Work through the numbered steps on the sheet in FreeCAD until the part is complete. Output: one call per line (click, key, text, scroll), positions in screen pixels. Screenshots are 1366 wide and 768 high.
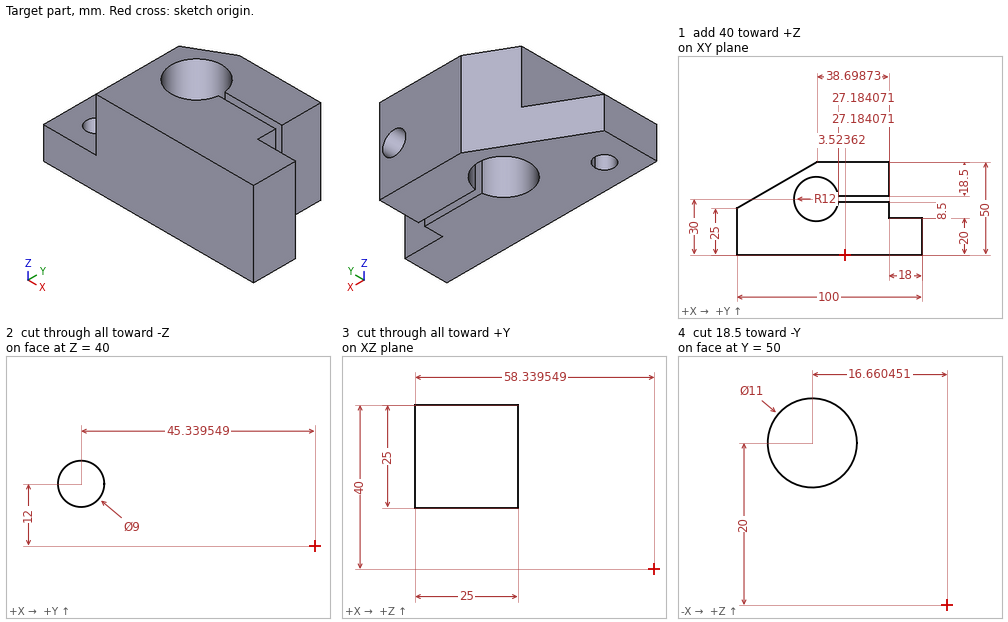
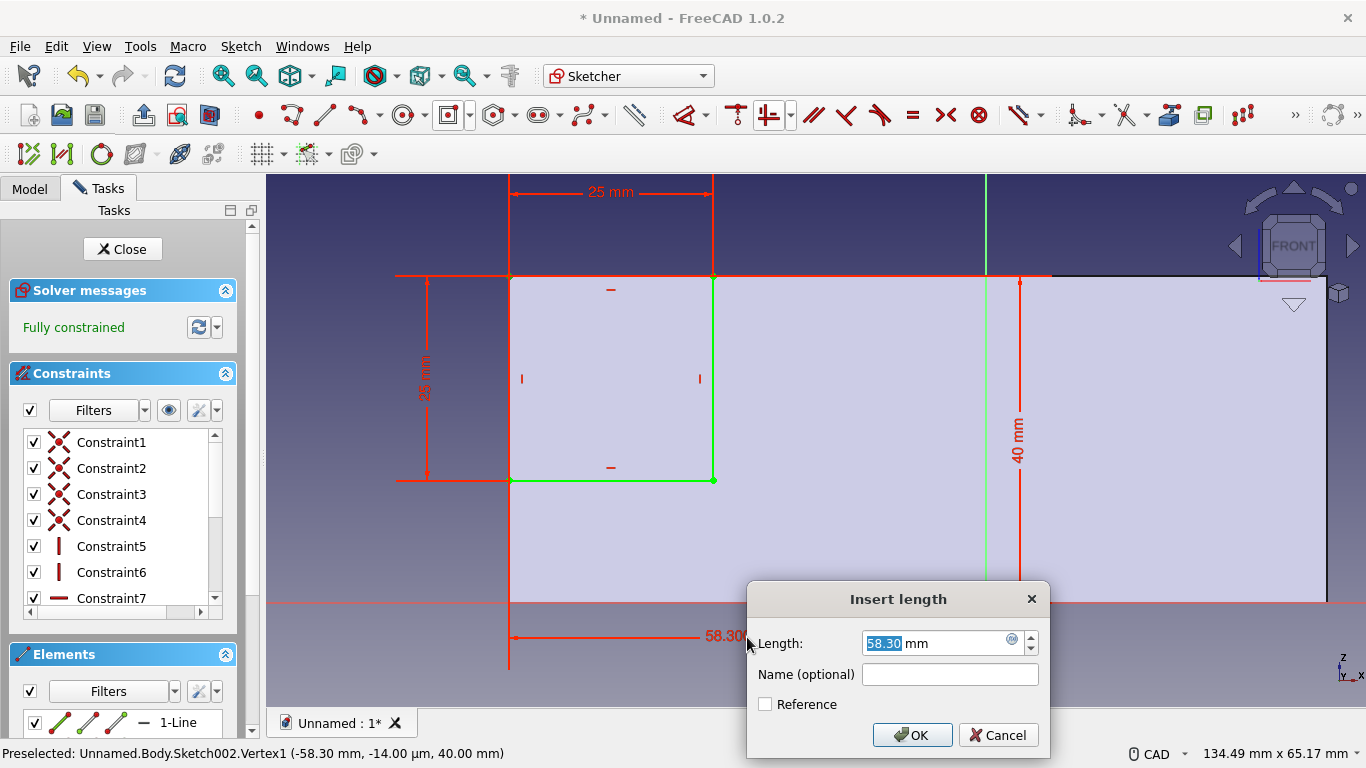
text(58.339549)
key(Return)
key(Escape)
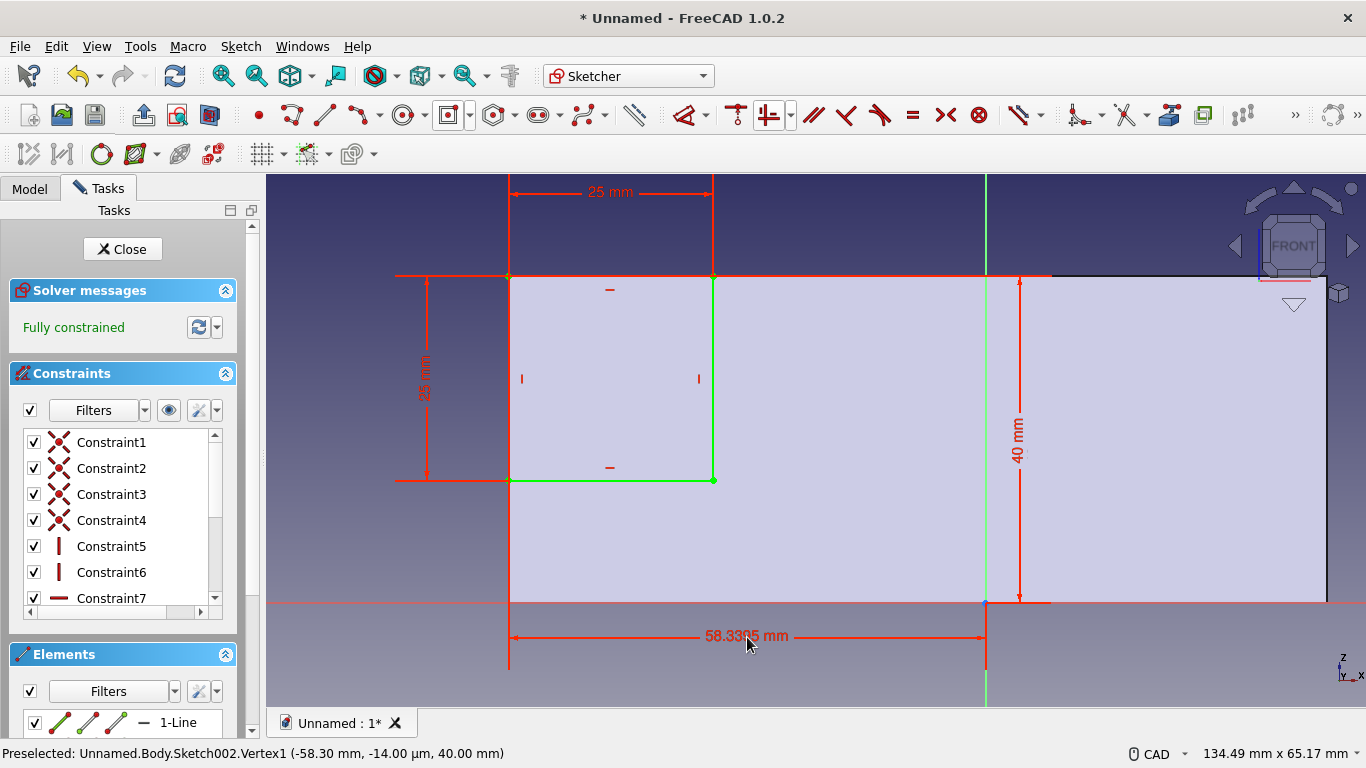
click(123, 249)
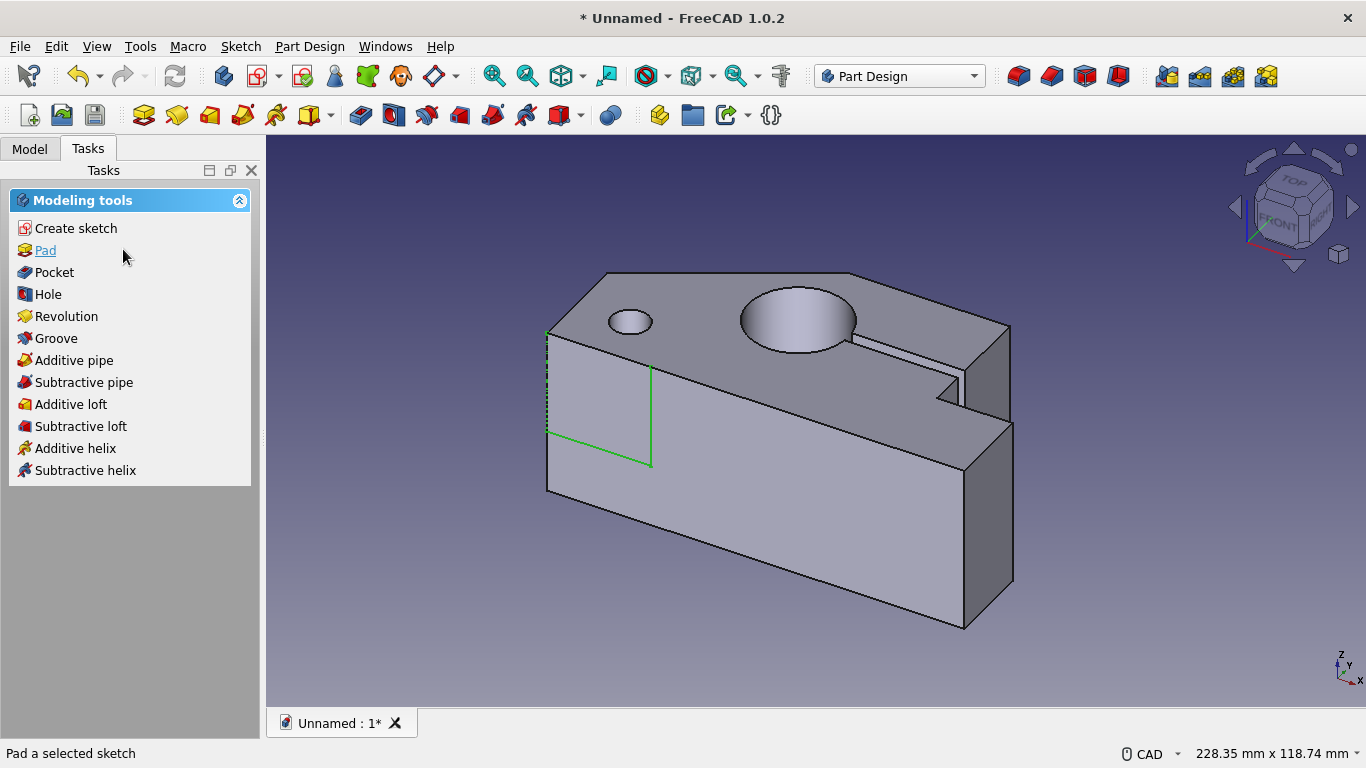
click(361, 116)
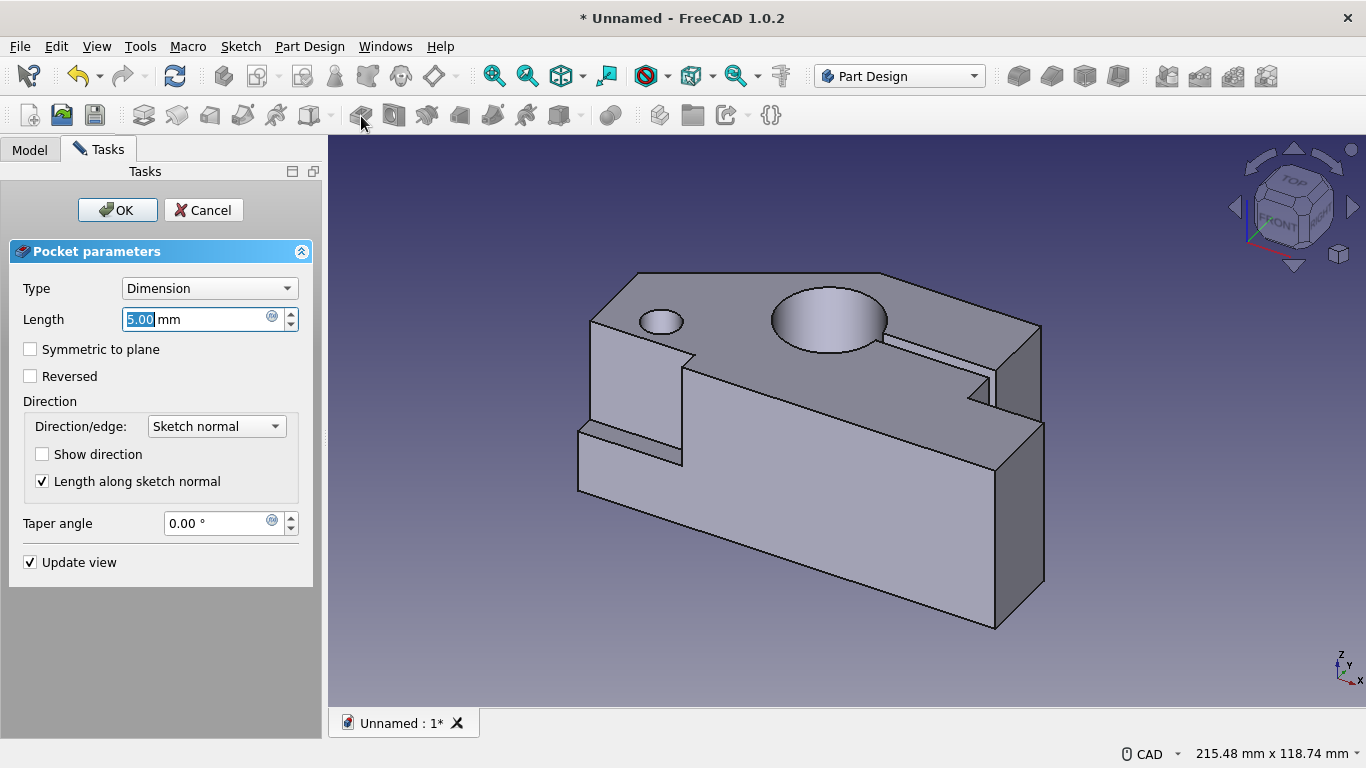
click(210, 288)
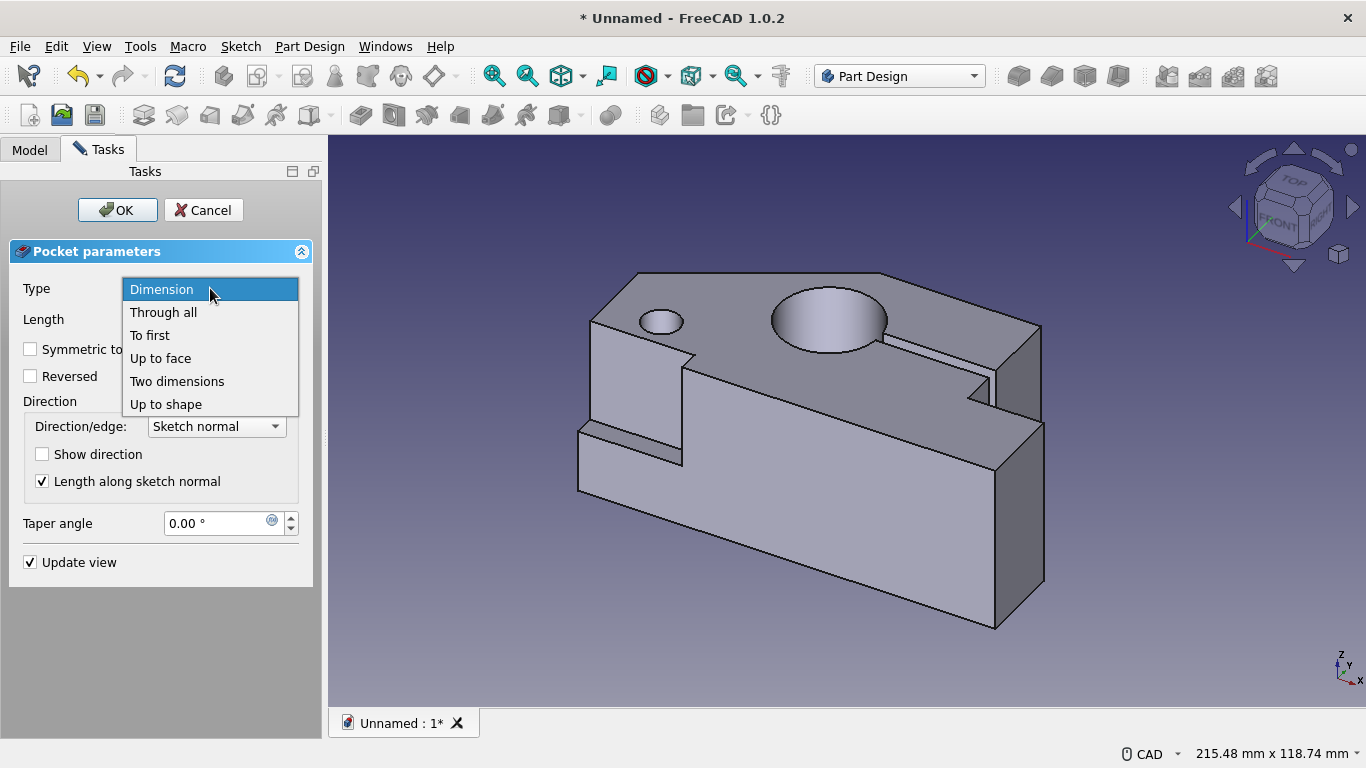
click(208, 312)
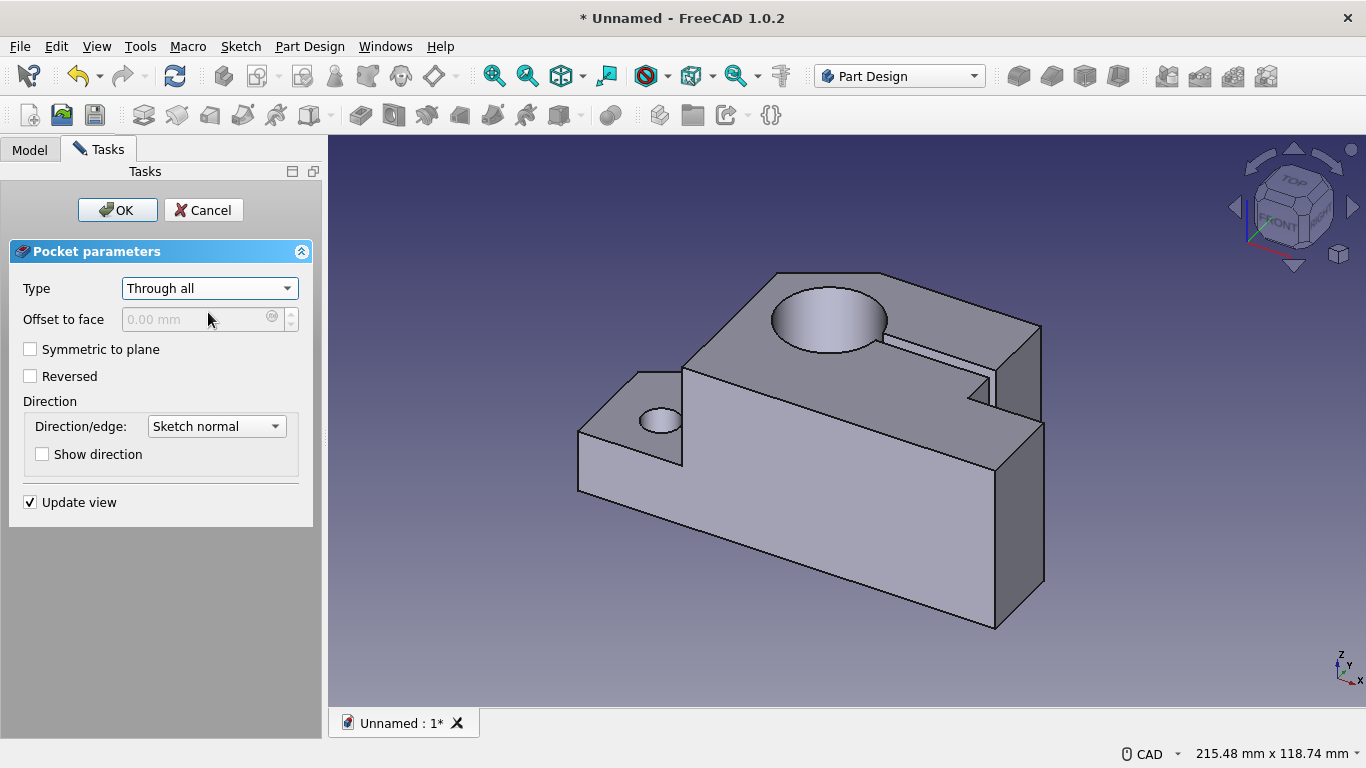
click(118, 210)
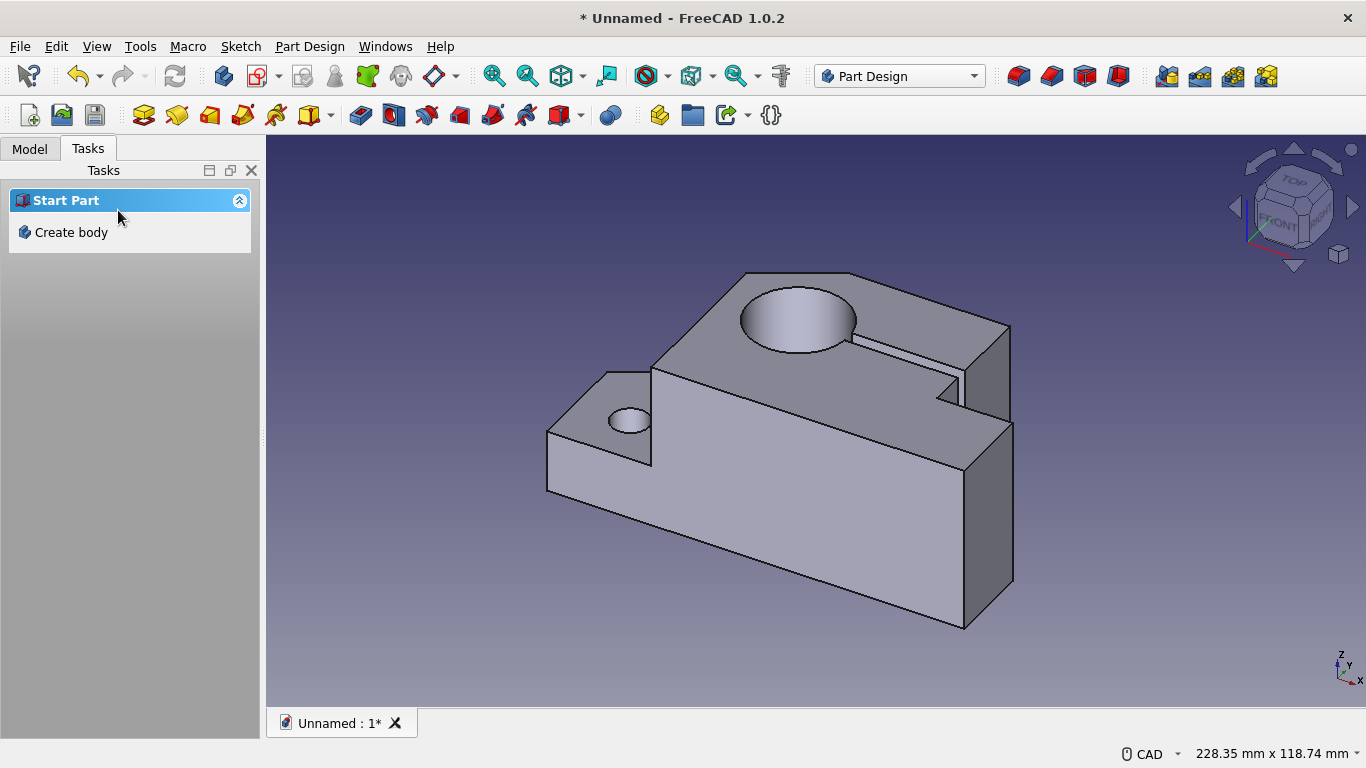
key(4)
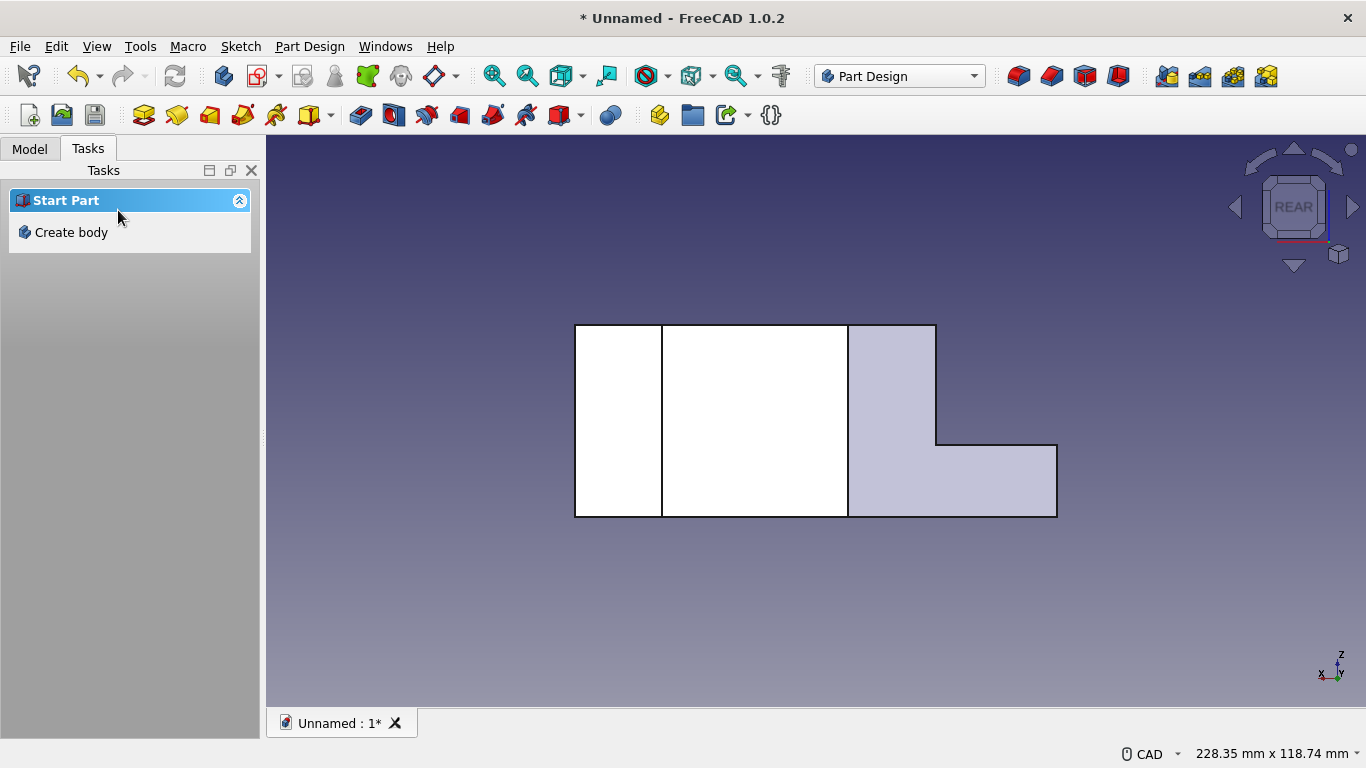
click(495, 76)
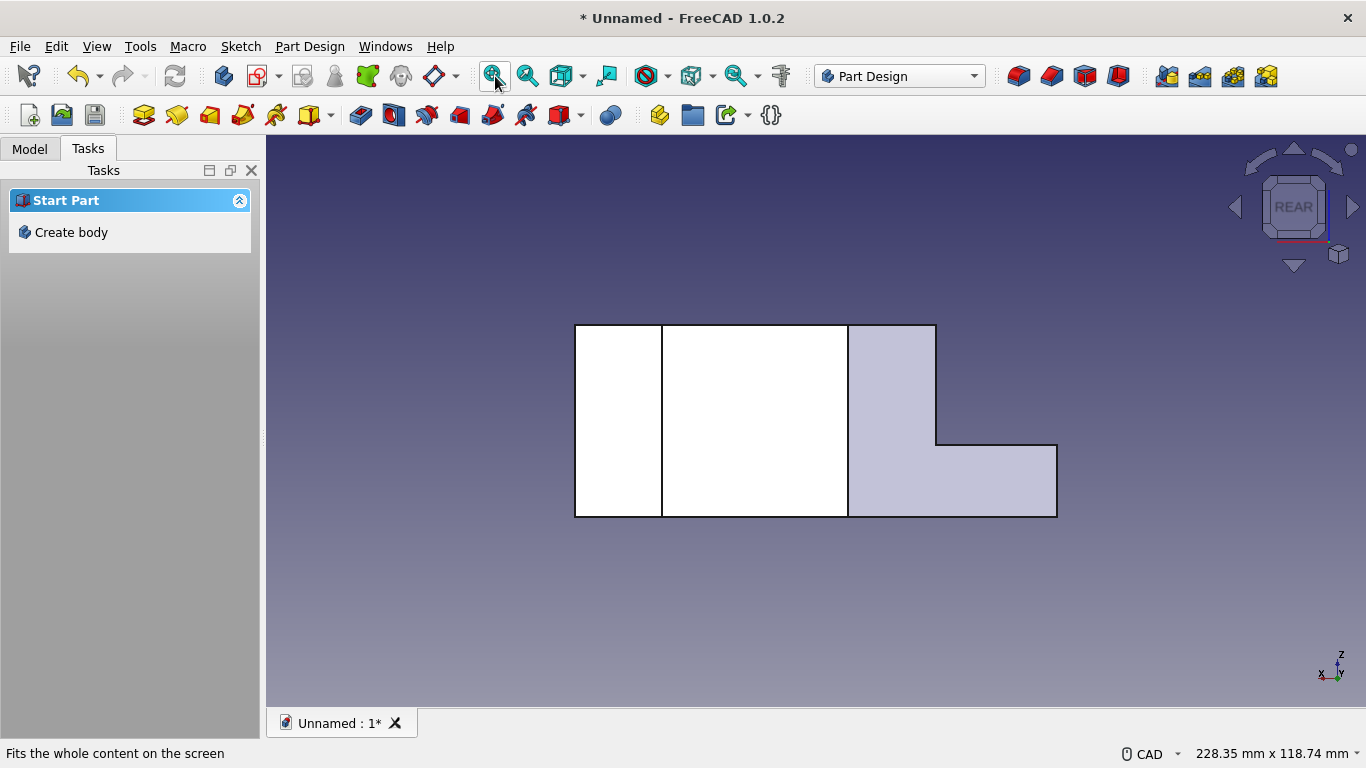
click(755, 420)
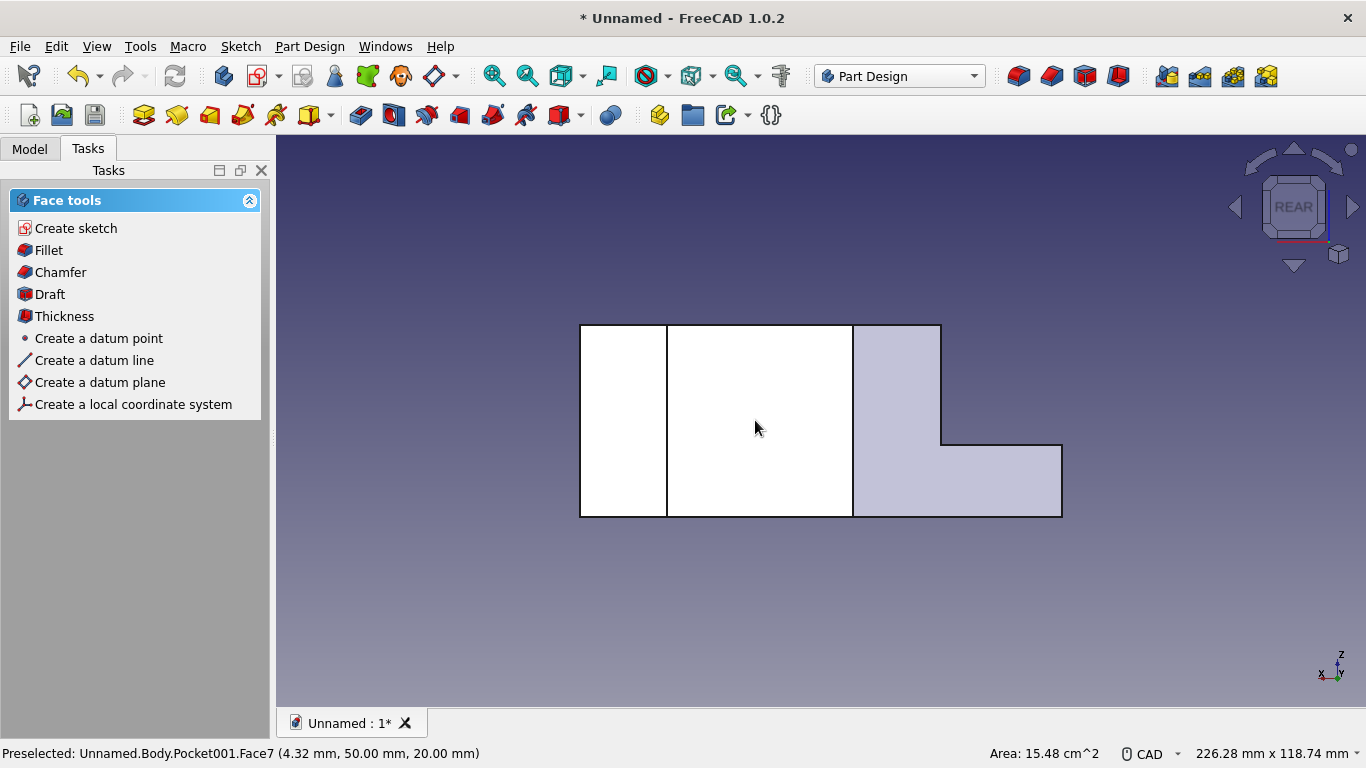
click(256, 76)